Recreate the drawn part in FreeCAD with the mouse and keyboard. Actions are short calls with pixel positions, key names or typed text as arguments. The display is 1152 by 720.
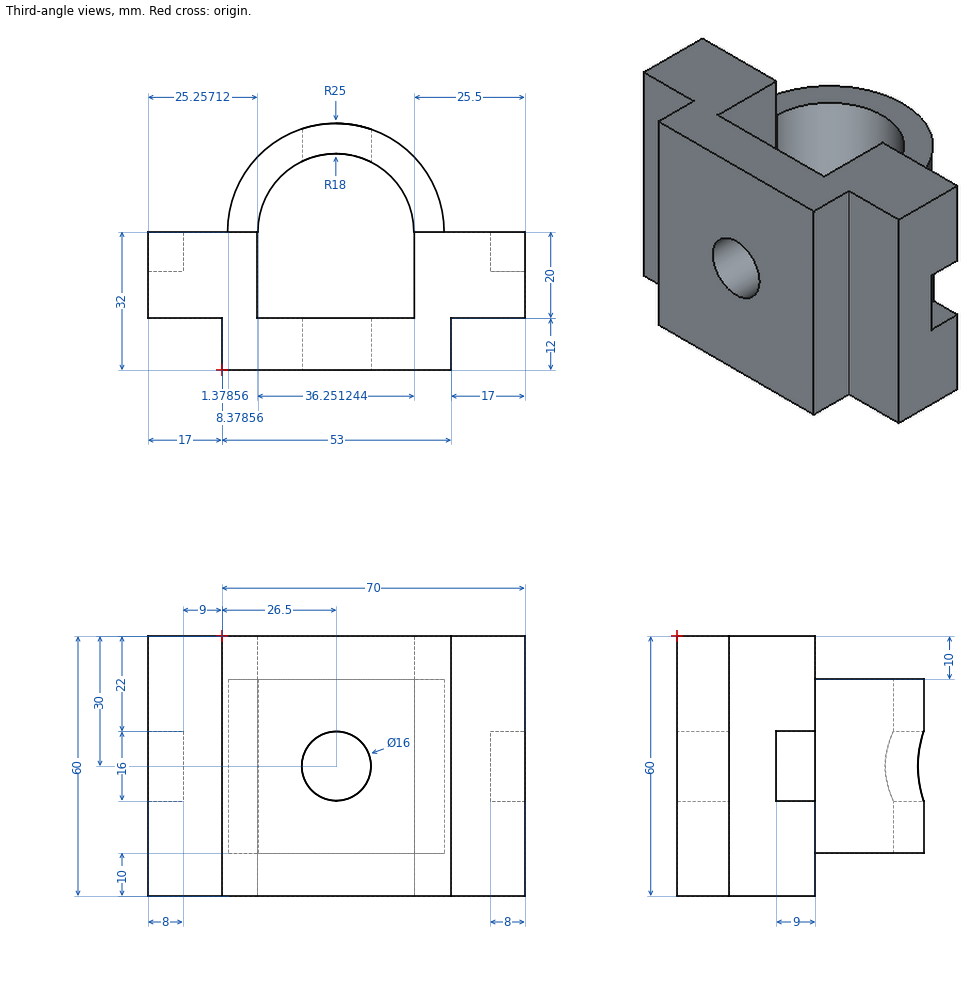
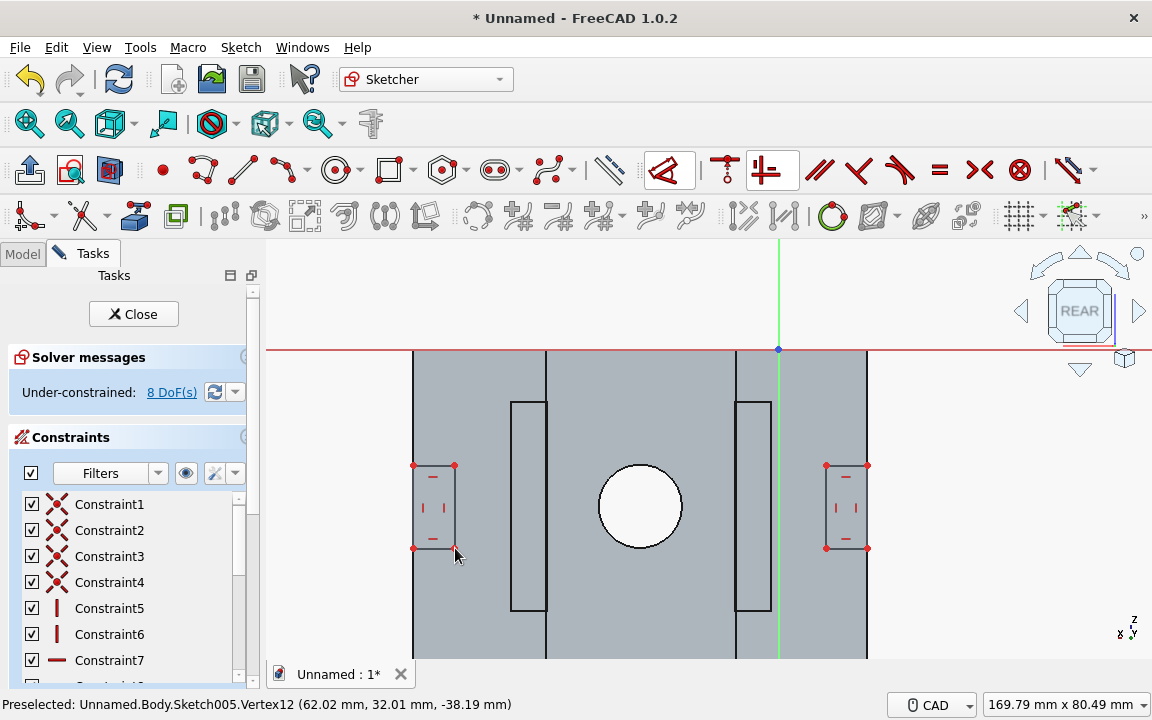
click(838, 549)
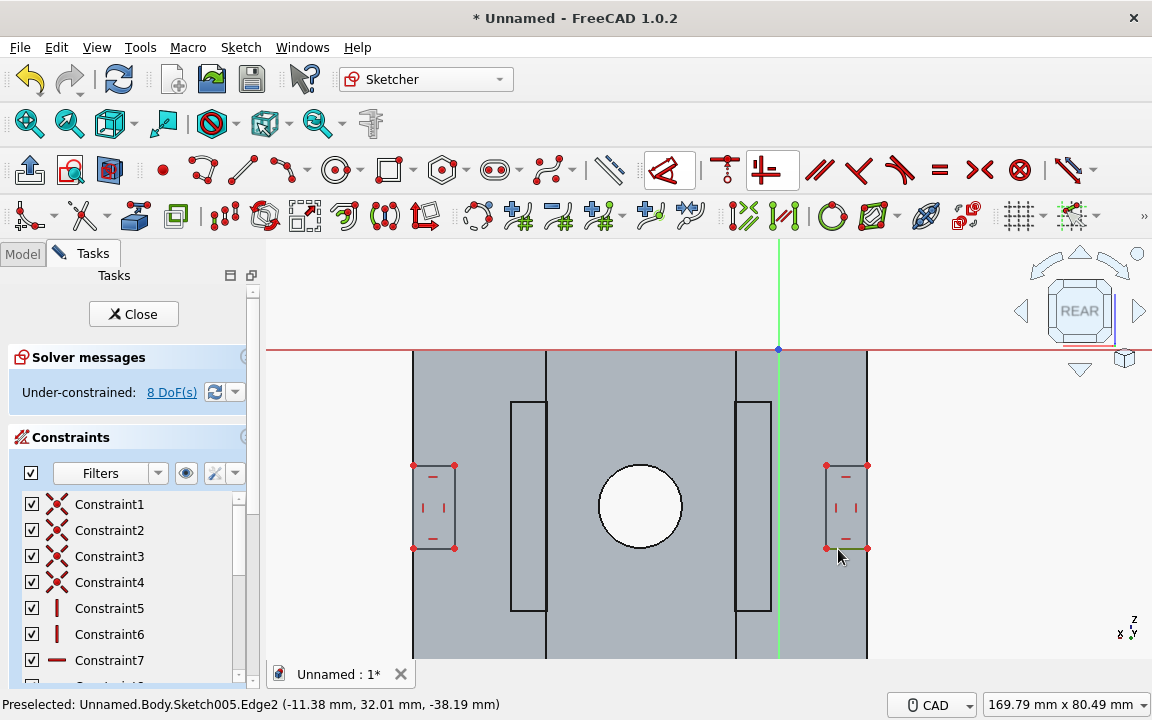
key(l)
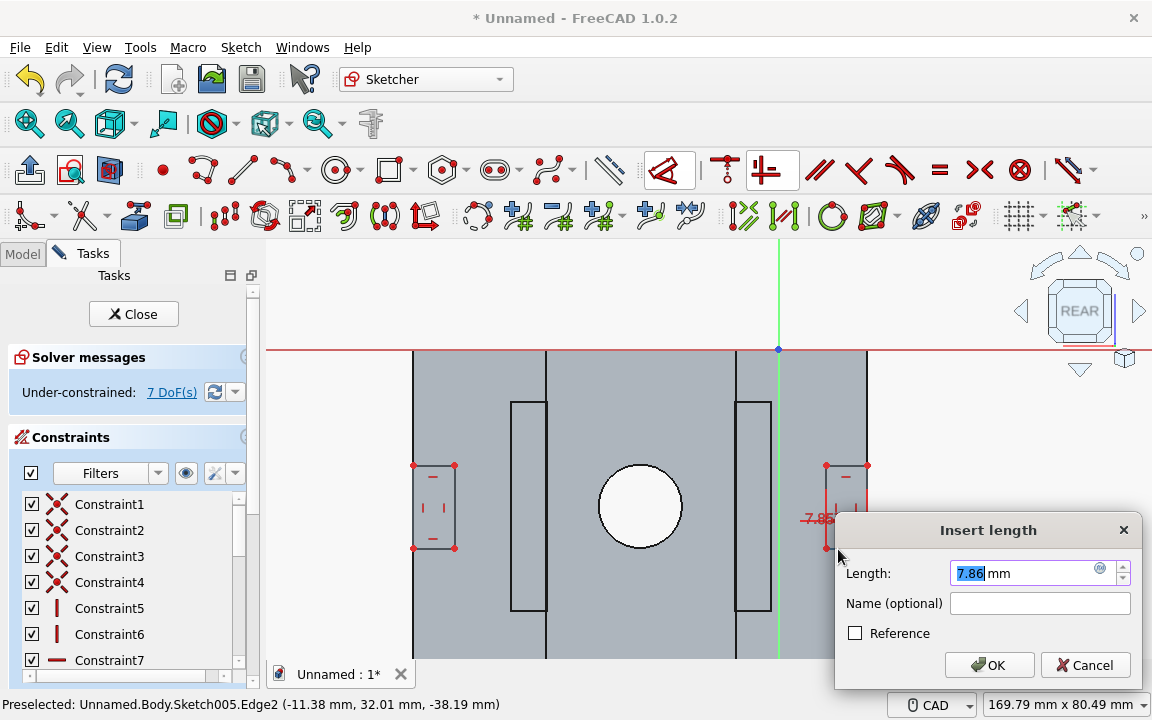
text(8)
key(Return)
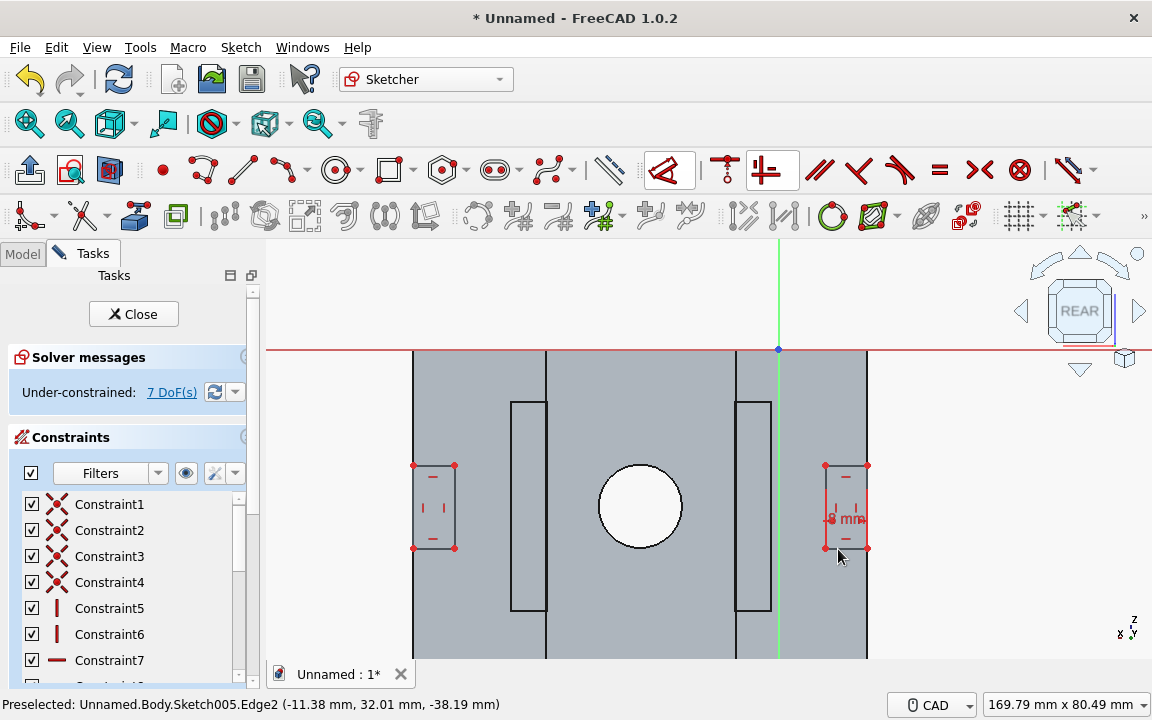
click(426, 549)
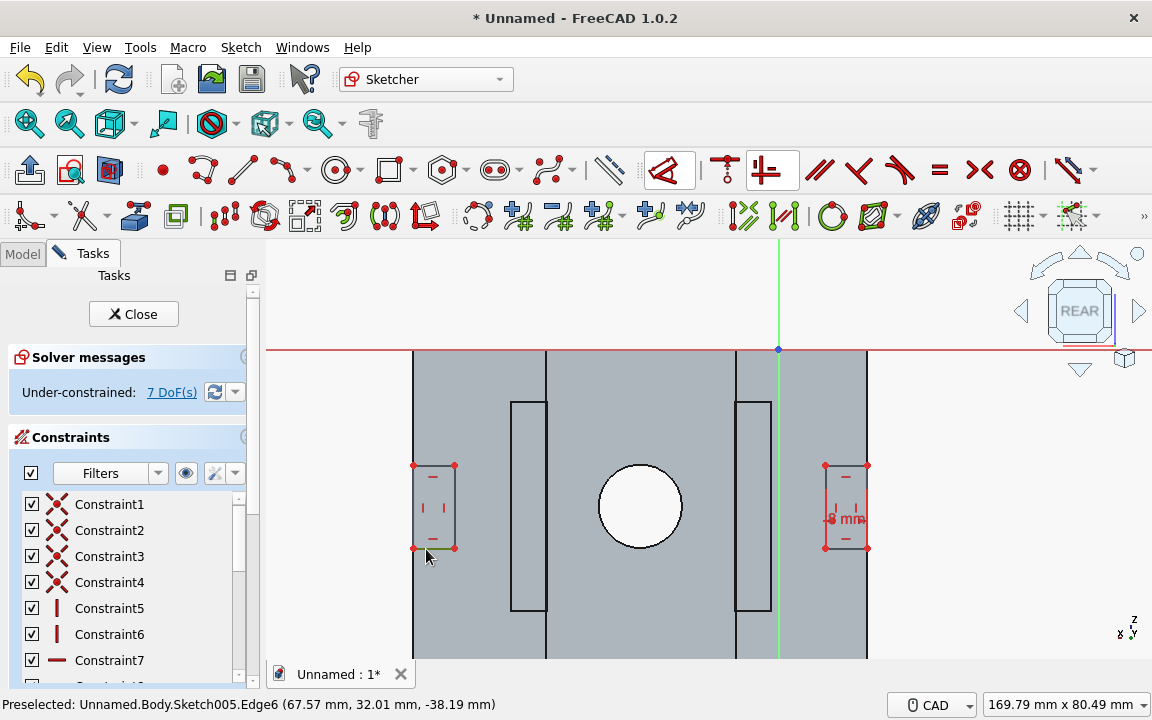
key(l)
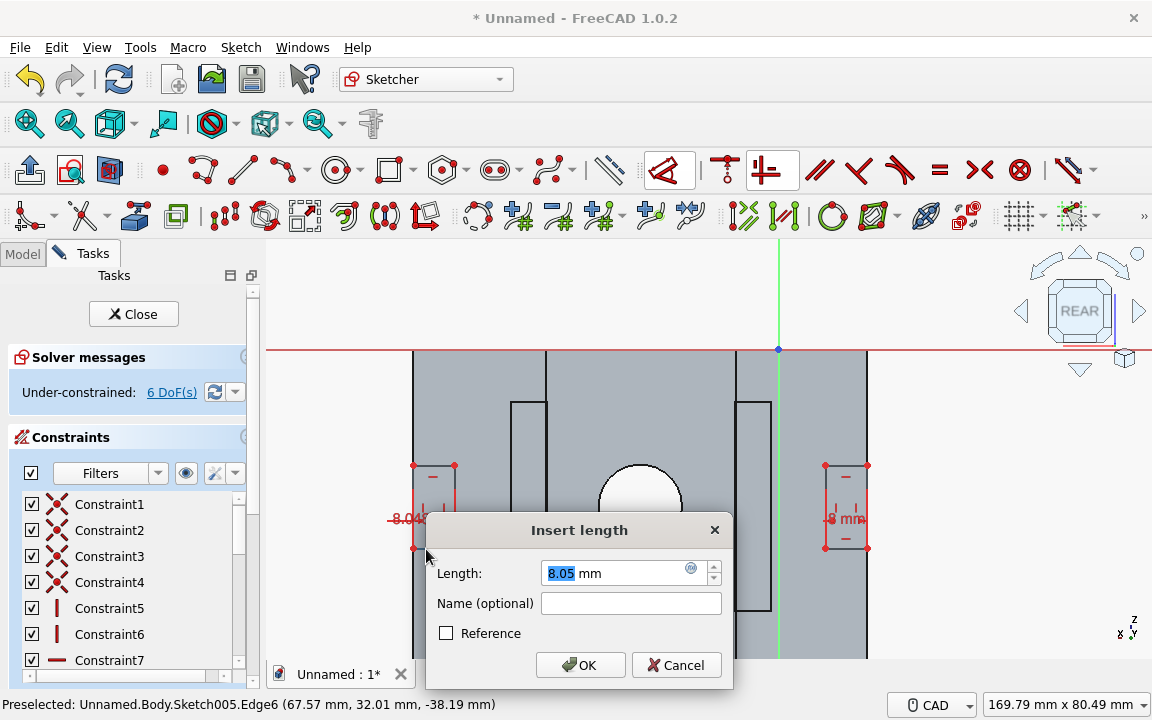
text(8)
key(Return)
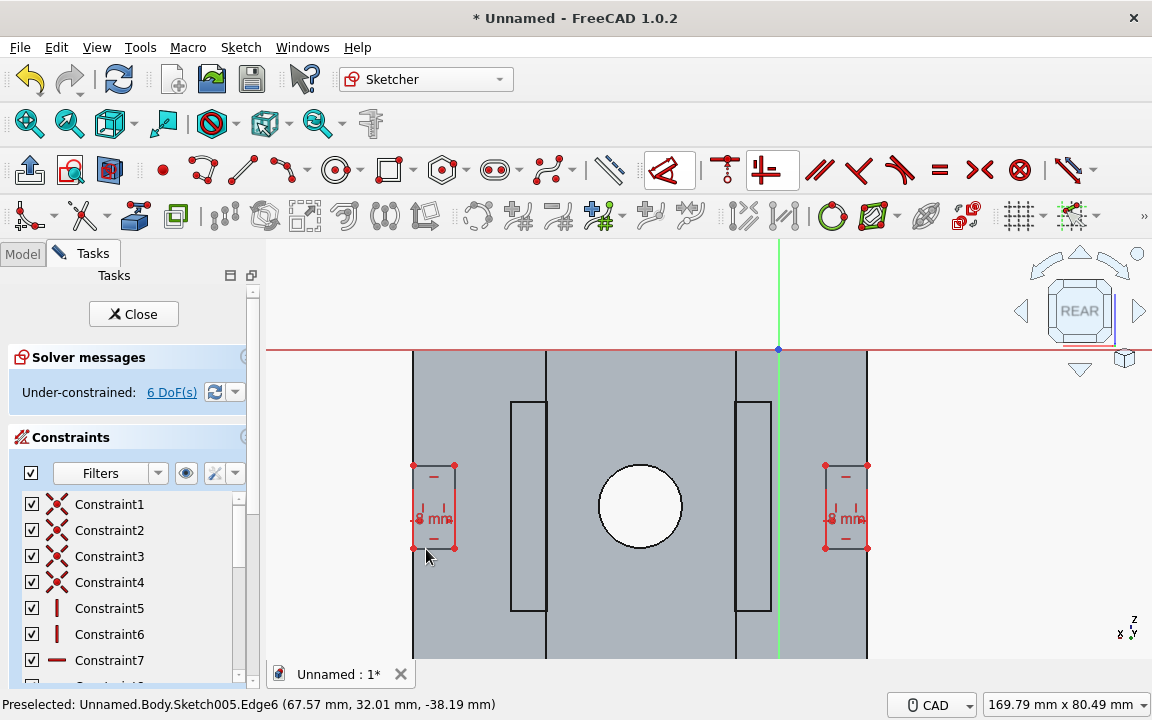
click(826, 491)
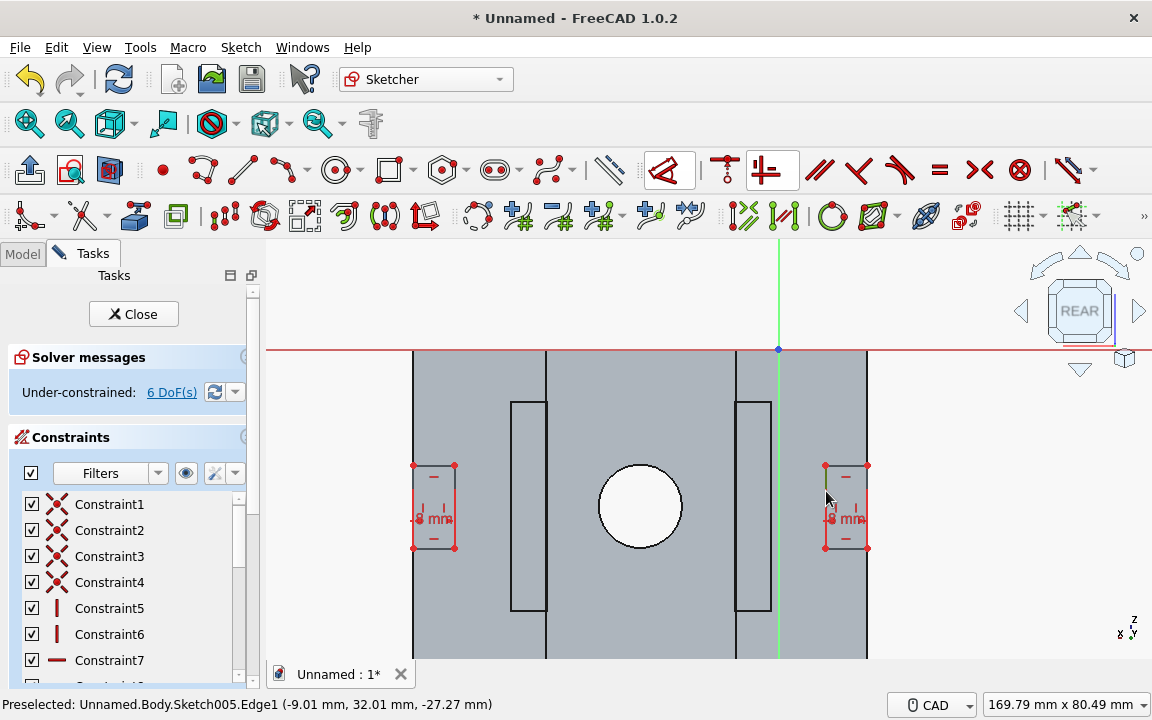
key(i)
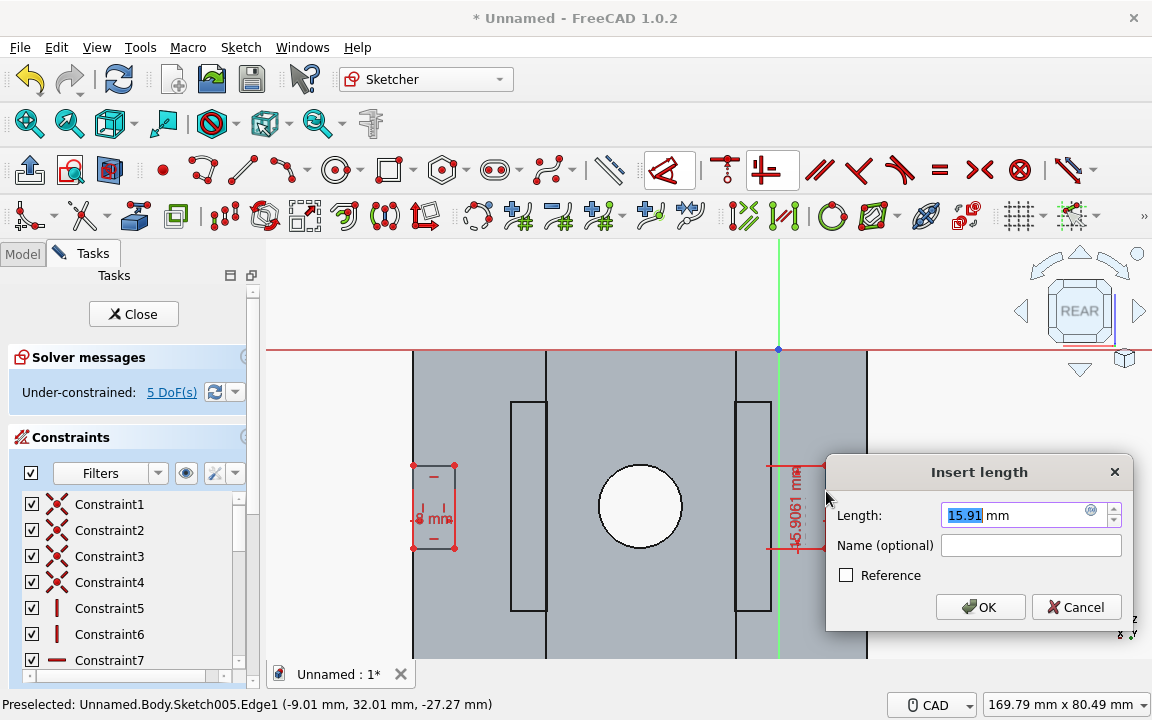
text(16)
key(Return)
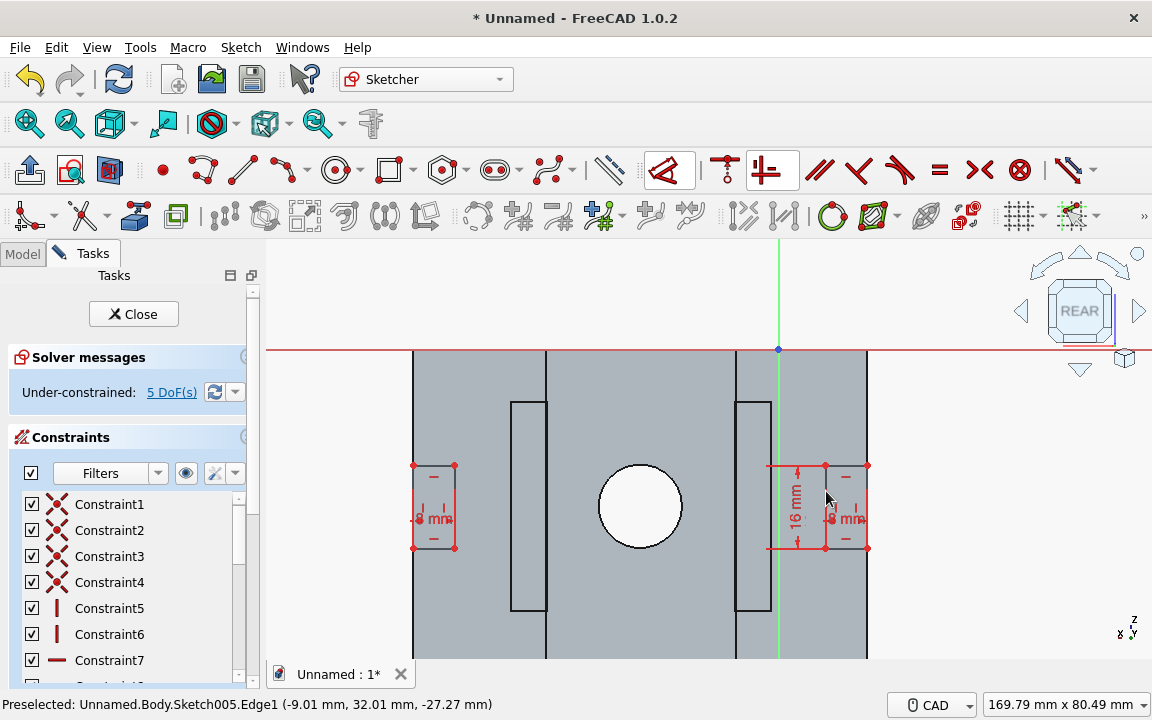
click(413, 491)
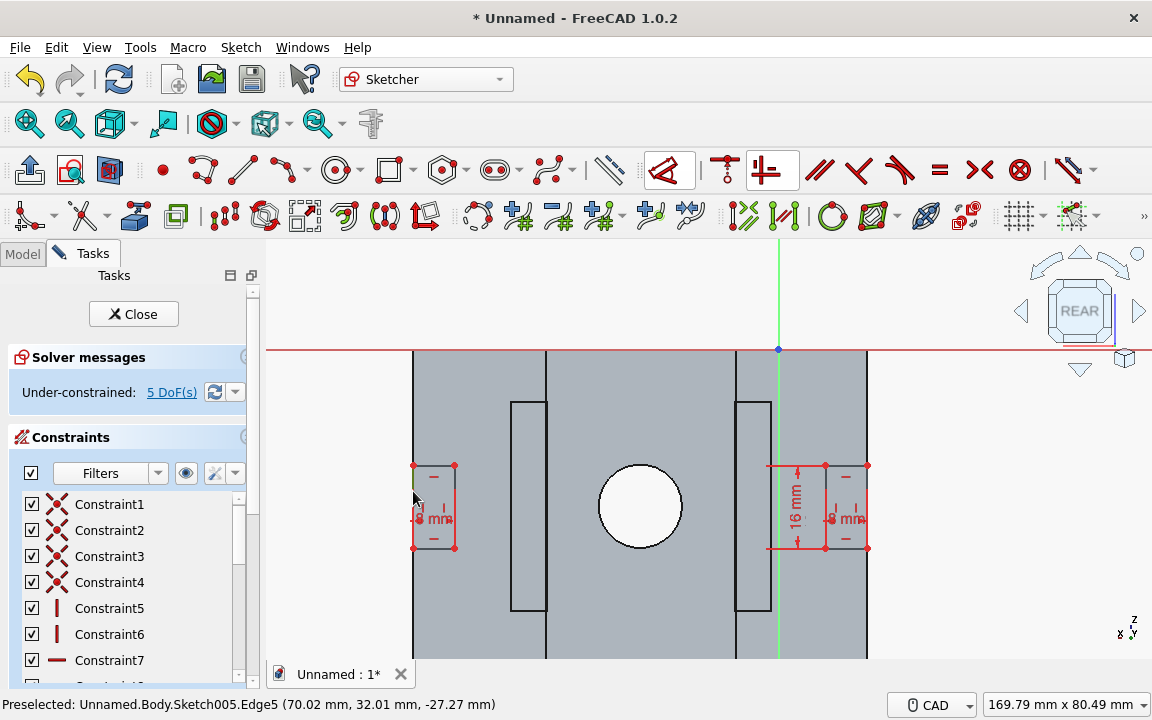
key(i)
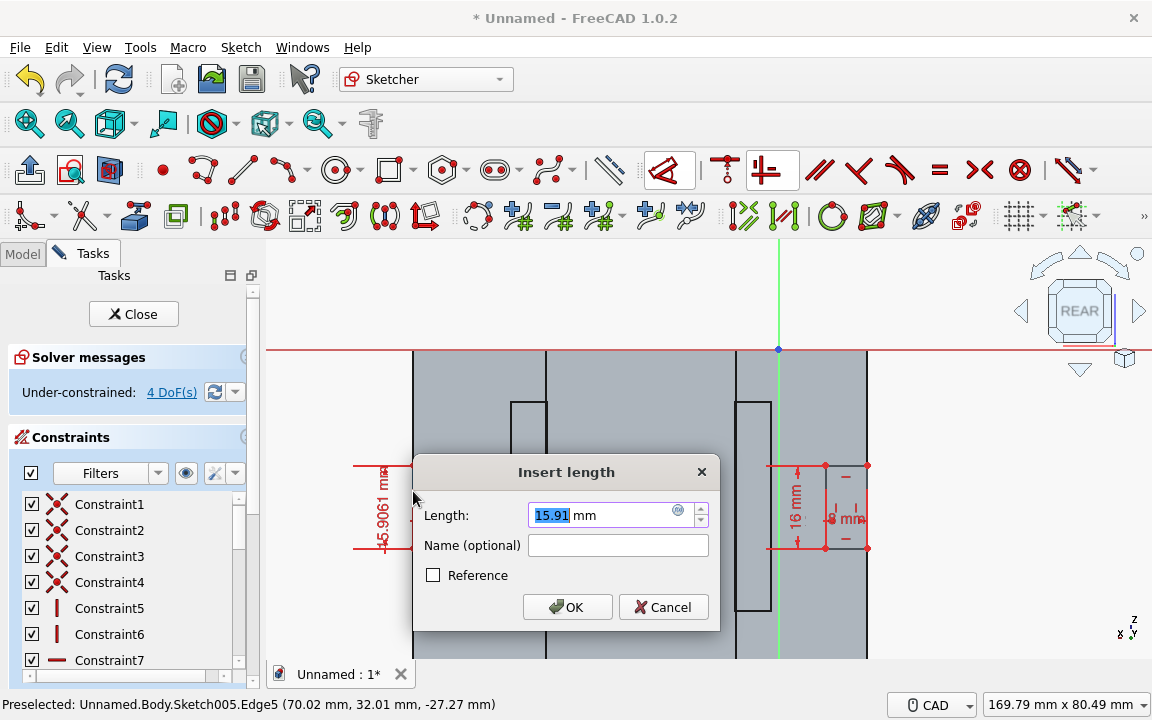
text(16)
key(Return)